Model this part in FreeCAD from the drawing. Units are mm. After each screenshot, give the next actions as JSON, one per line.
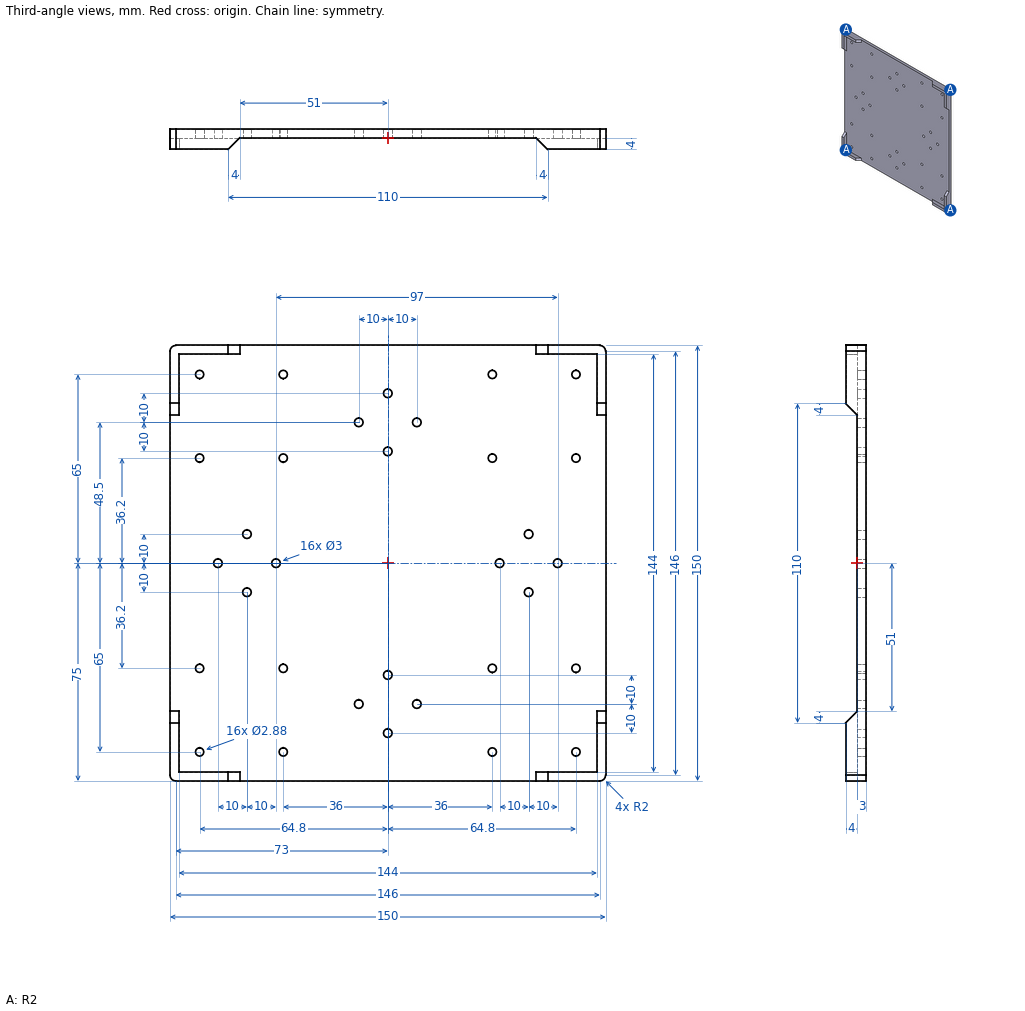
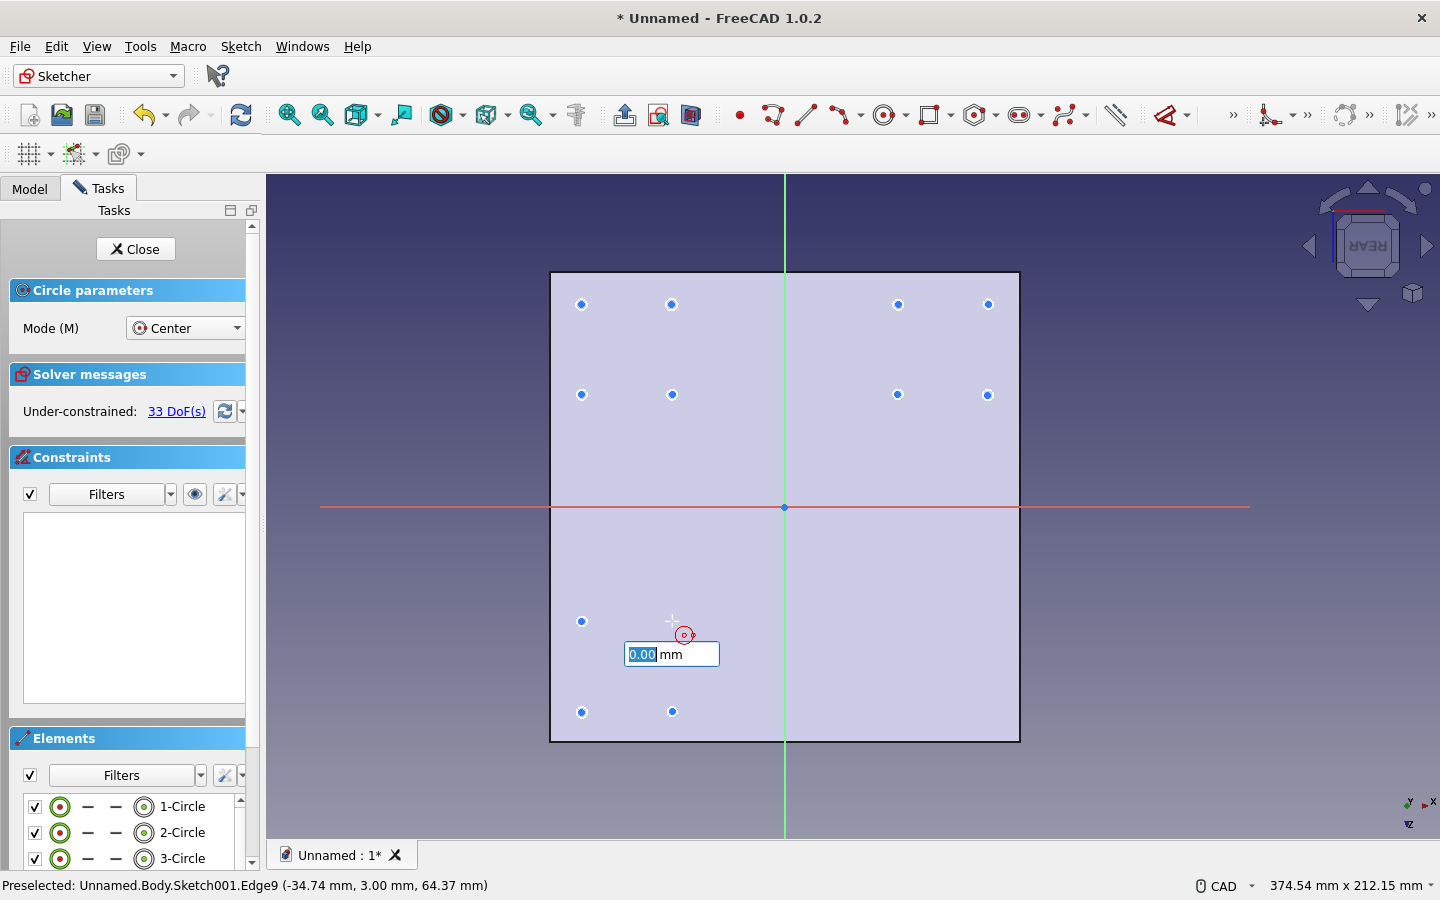
{"action": "scroll", "coordinate": [675, 617], "scroll_direction": "up", "scroll_amount": 7}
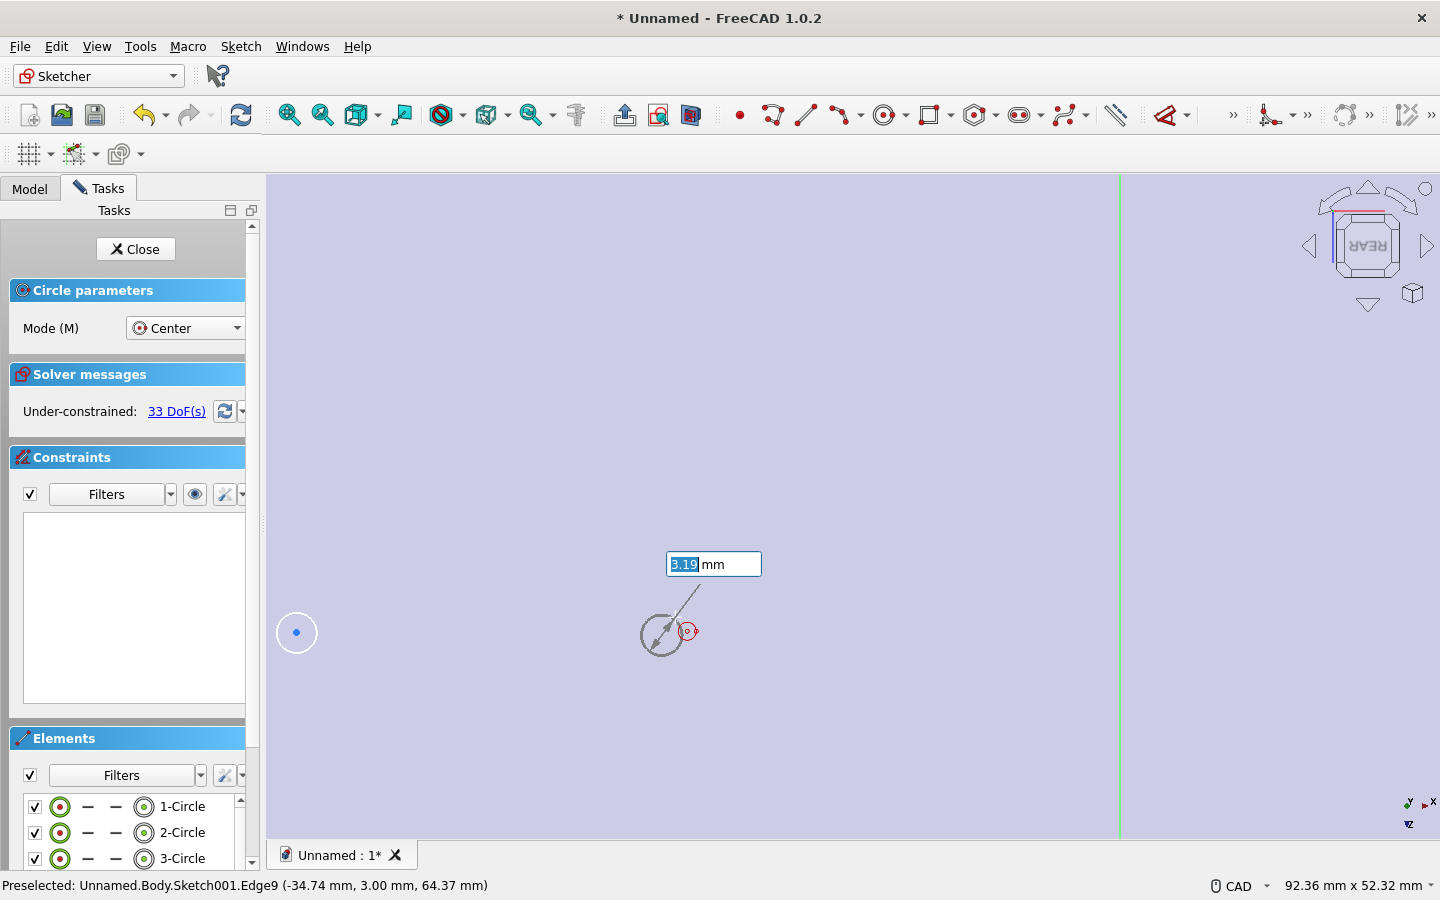
{"action": "left_click", "coordinate": [675, 617]}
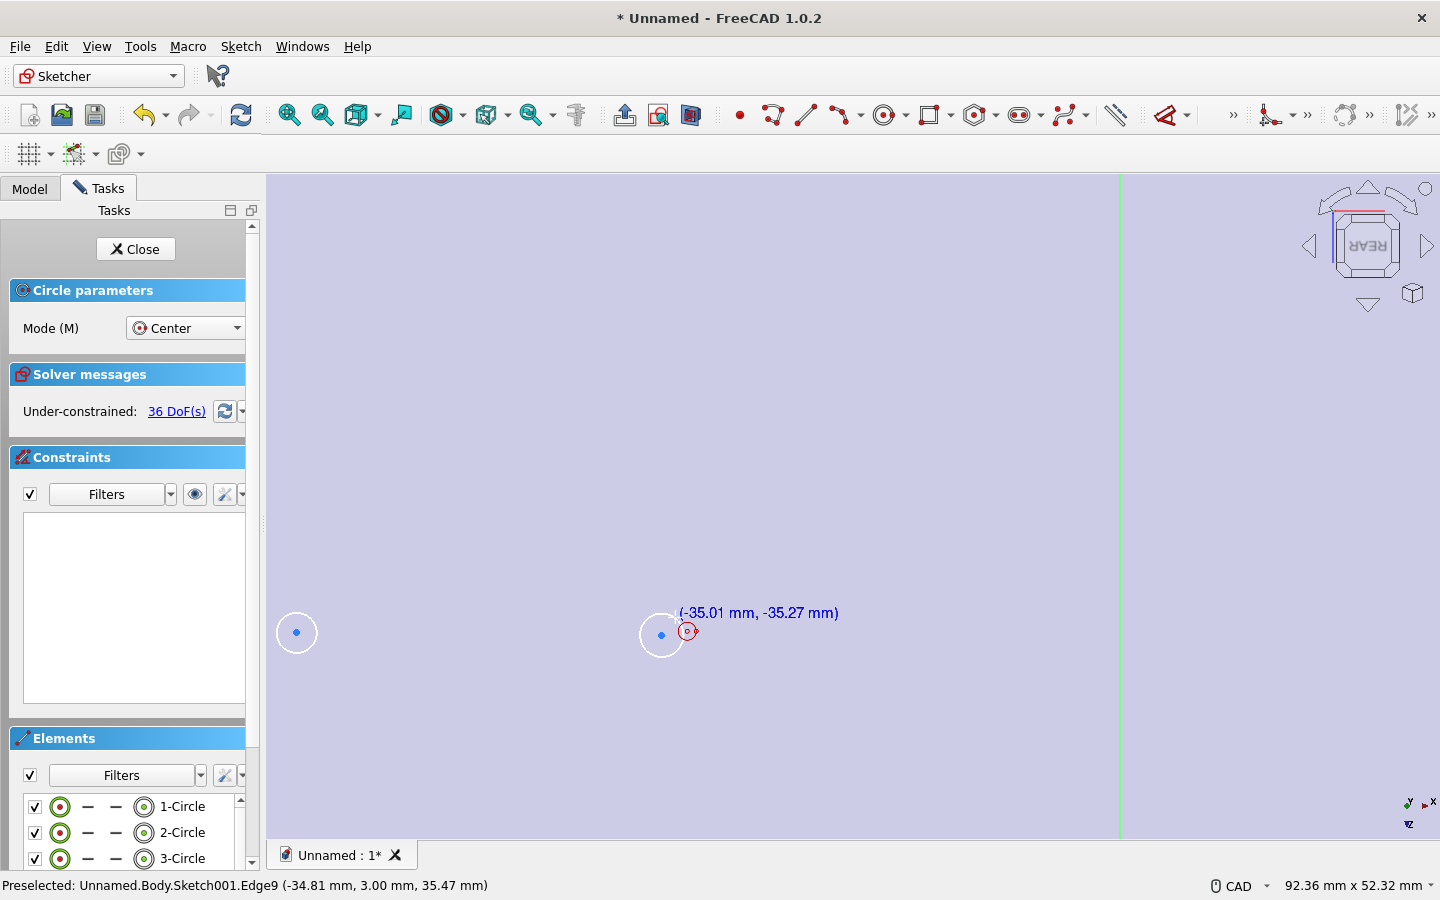
{"action": "scroll", "coordinate": [675, 617], "scroll_direction": "down", "scroll_amount": 7}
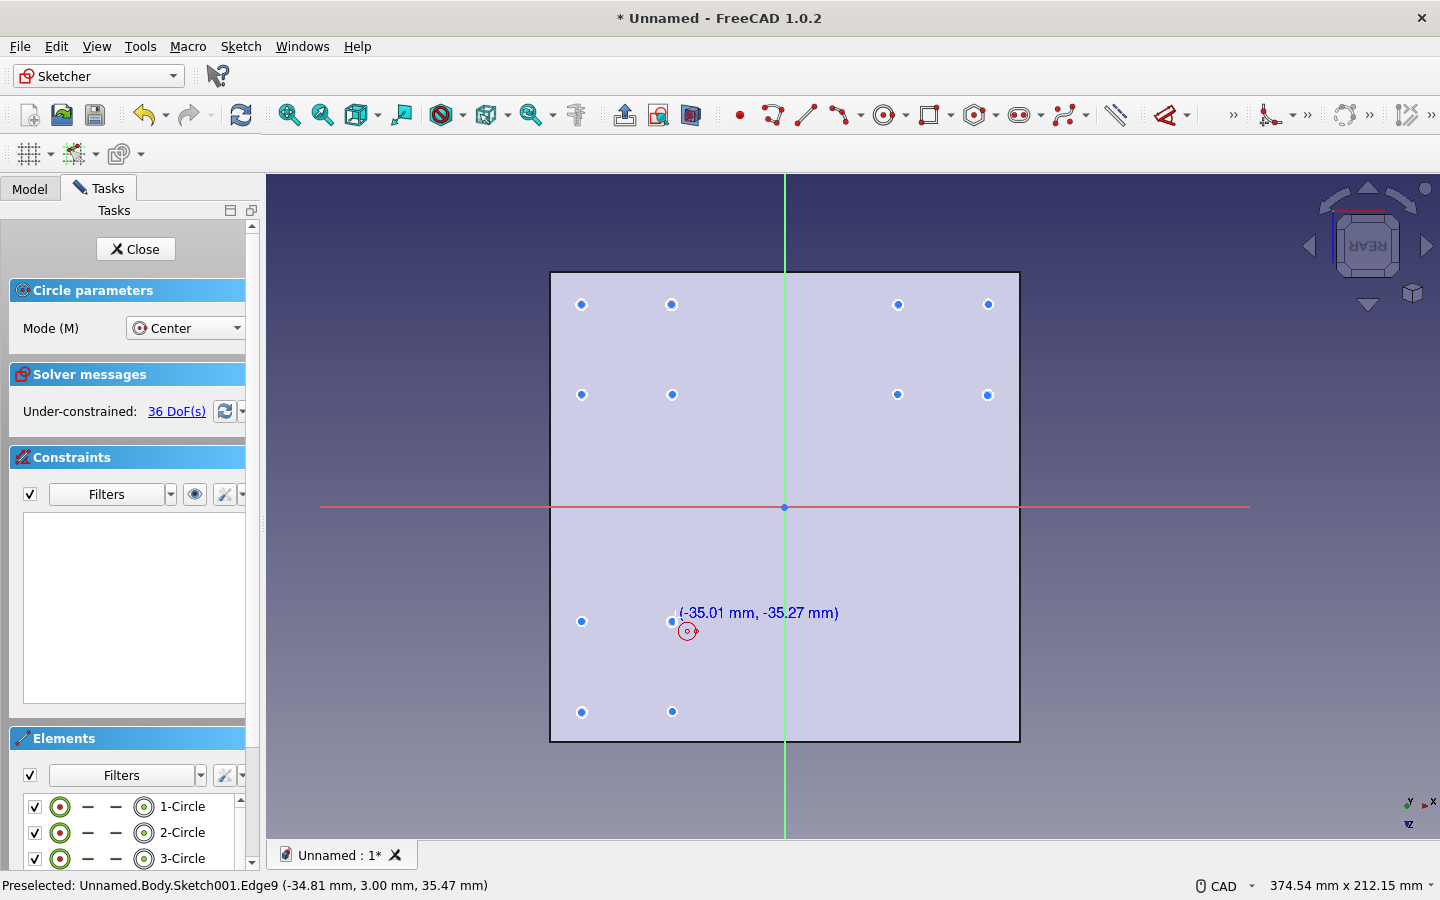
{"action": "scroll", "coordinate": [988, 711], "scroll_direction": "up", "scroll_amount": 9}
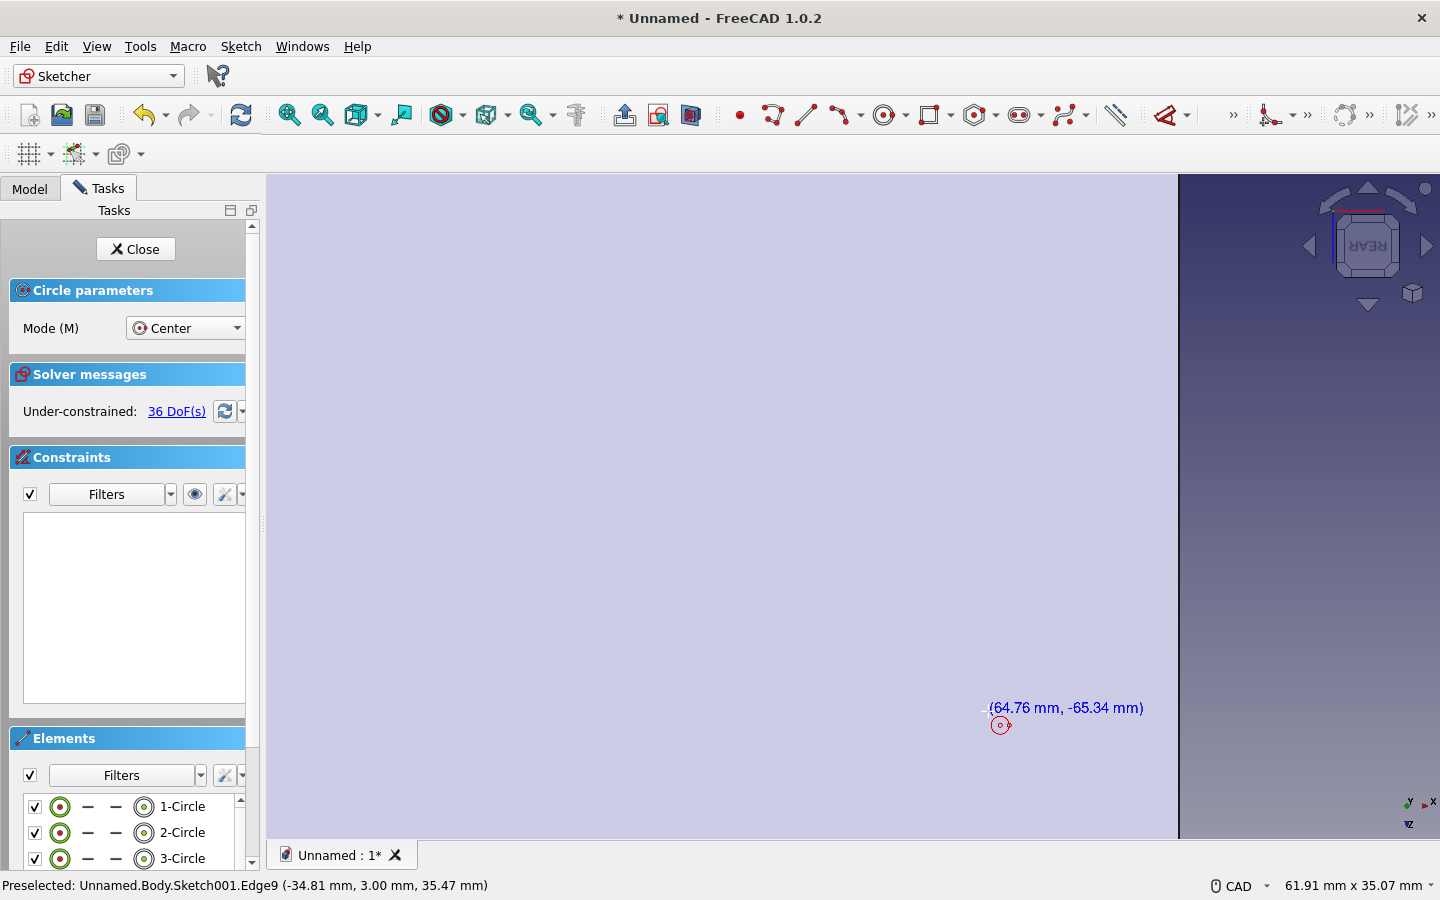
{"action": "scroll", "coordinate": [988, 711], "scroll_direction": "down", "scroll_amount": 9}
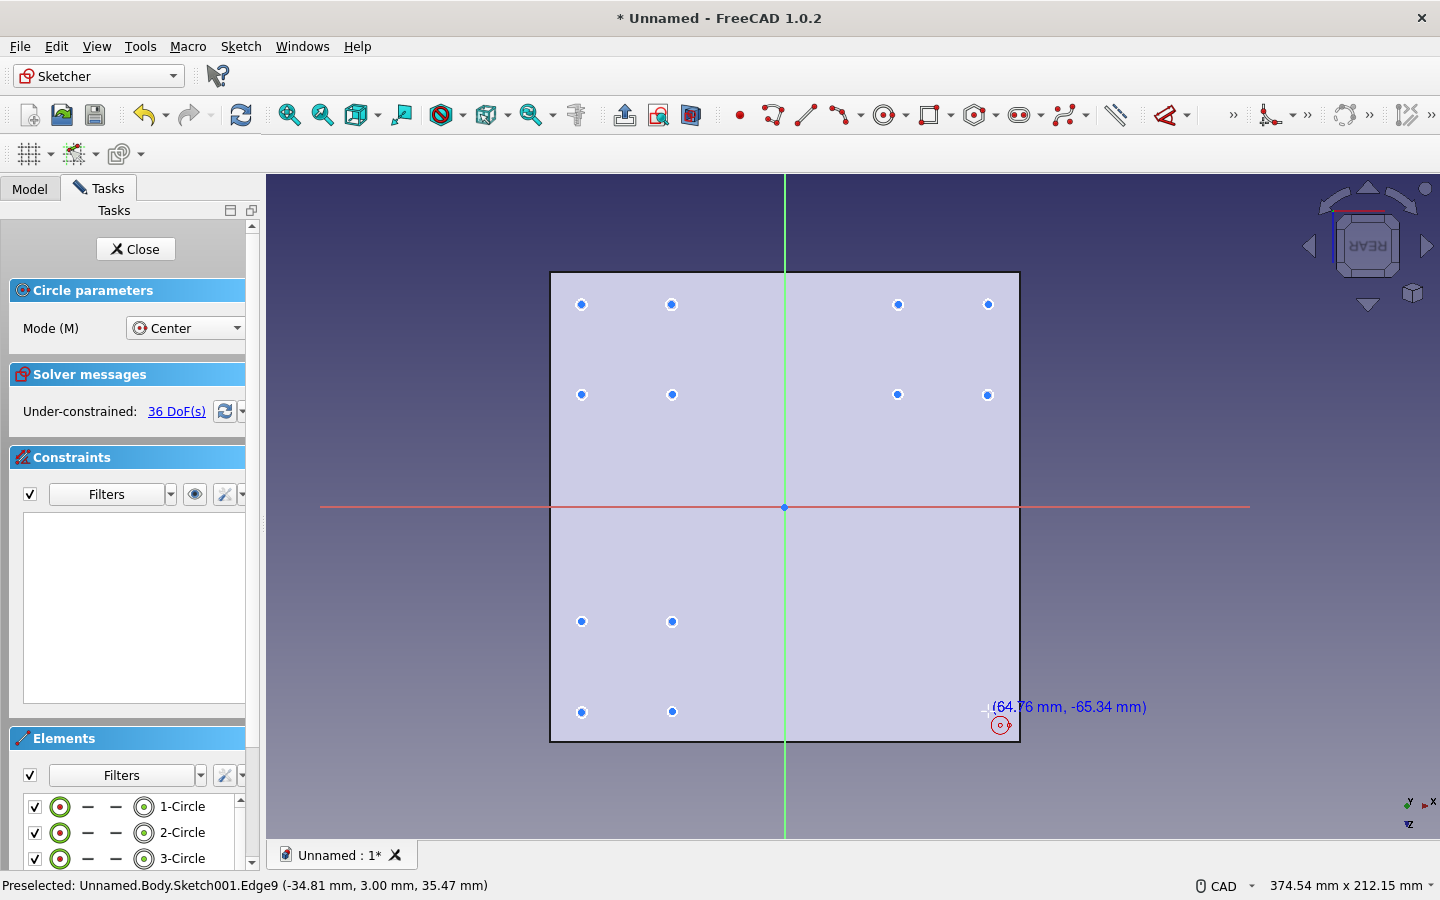
{"action": "left_click", "coordinate": [988, 711]}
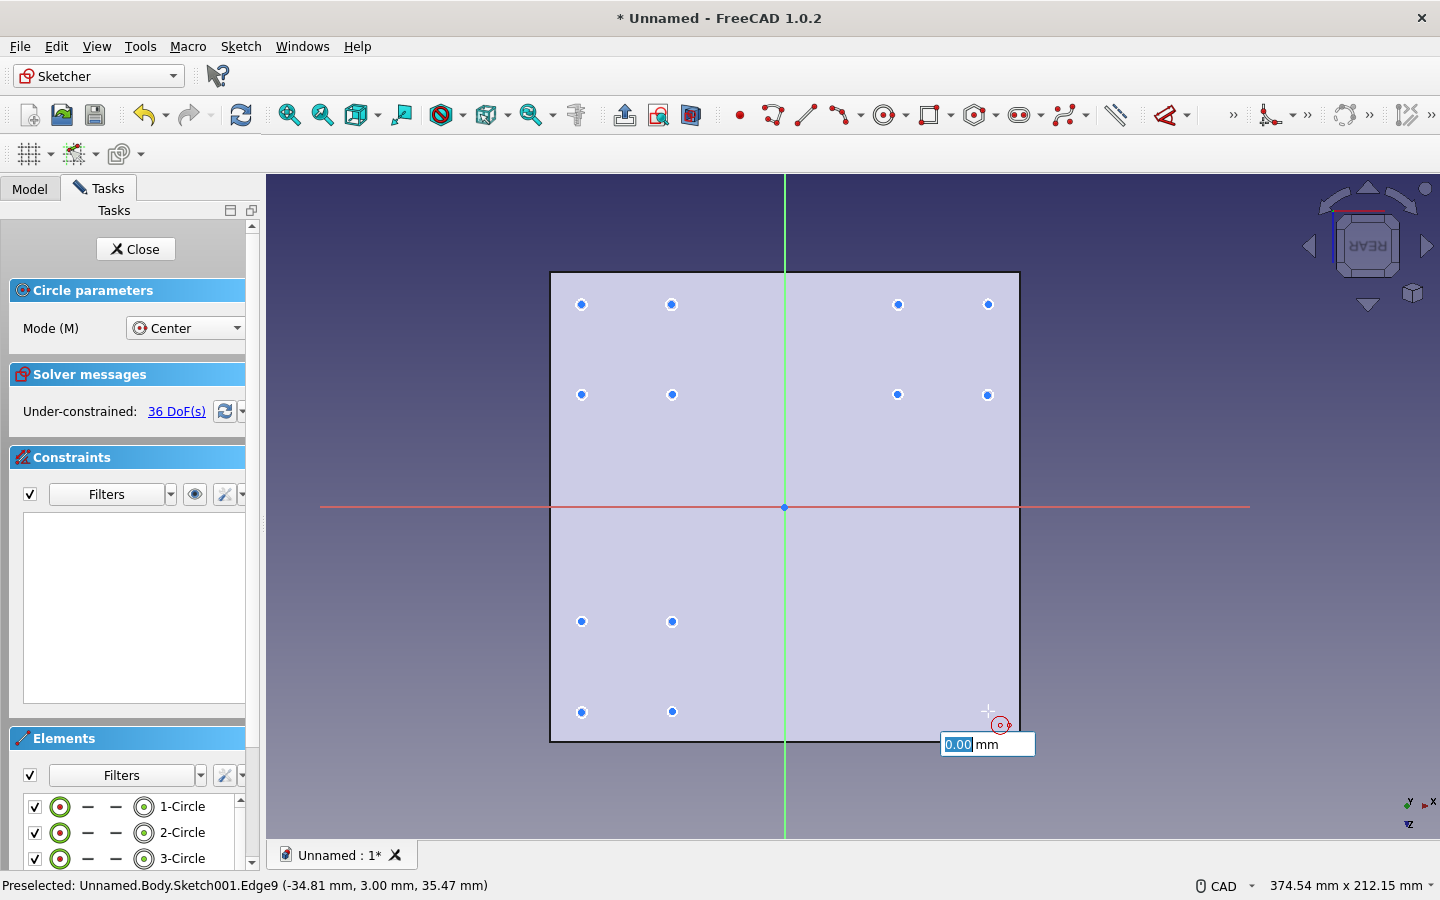
{"action": "scroll", "coordinate": [991, 708], "scroll_direction": "up", "scroll_amount": 7}